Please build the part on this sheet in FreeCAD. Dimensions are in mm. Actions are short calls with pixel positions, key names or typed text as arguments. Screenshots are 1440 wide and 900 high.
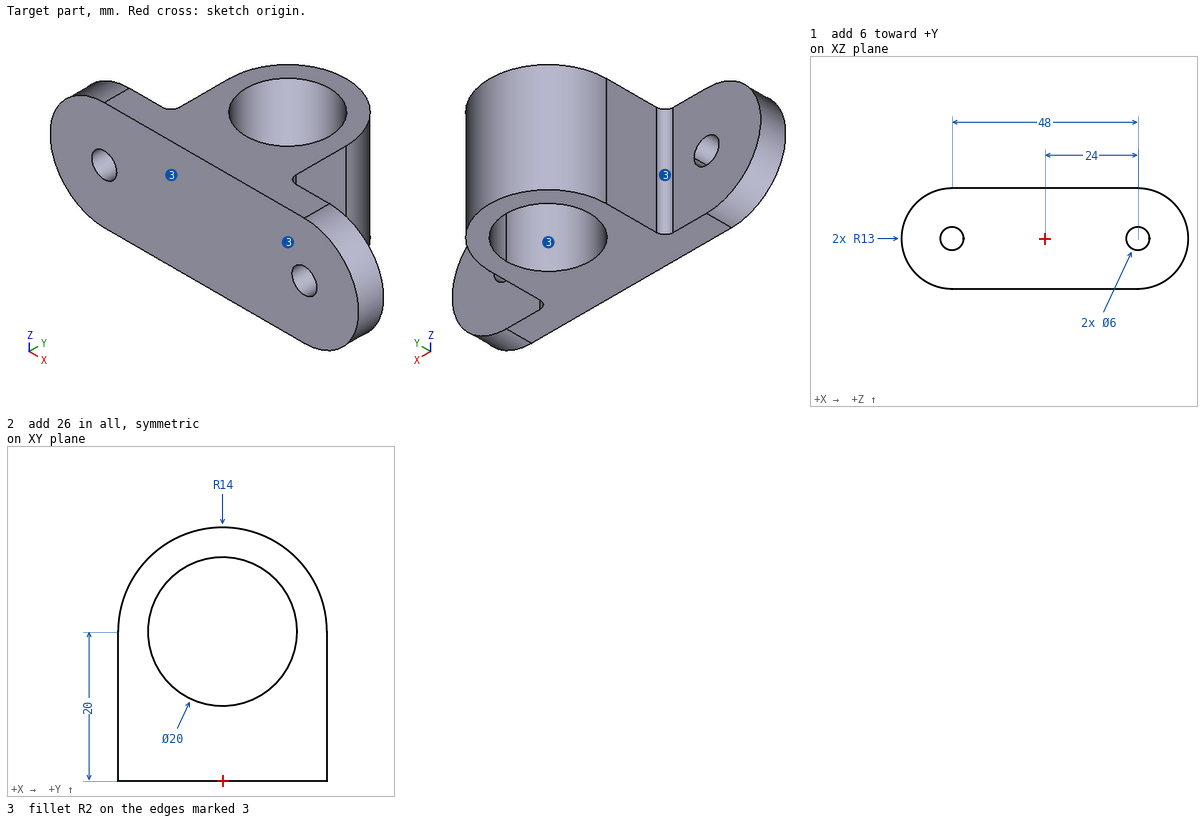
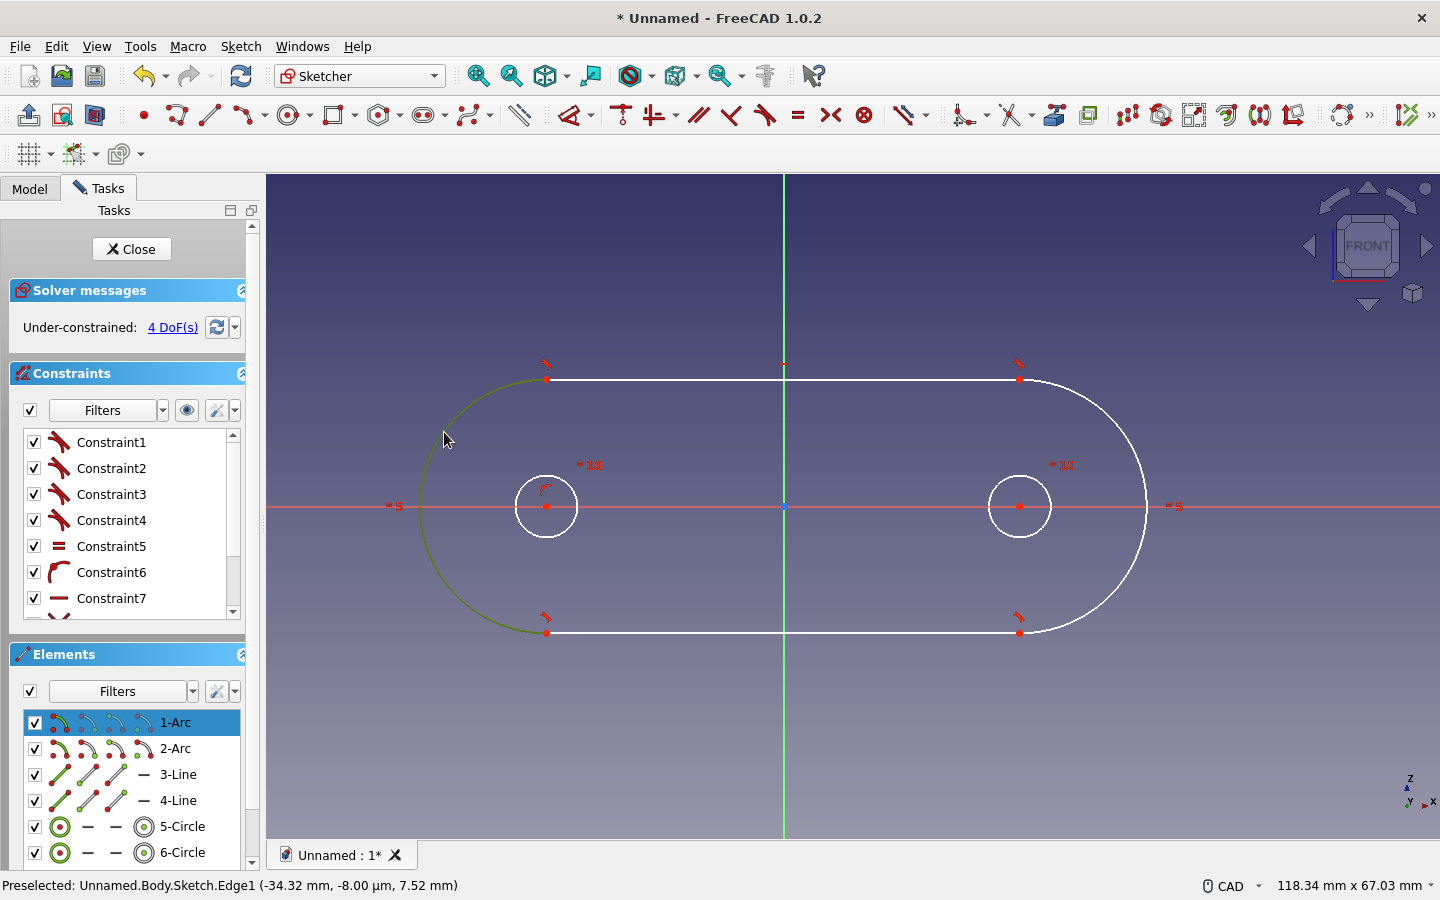
key(k)
key(r)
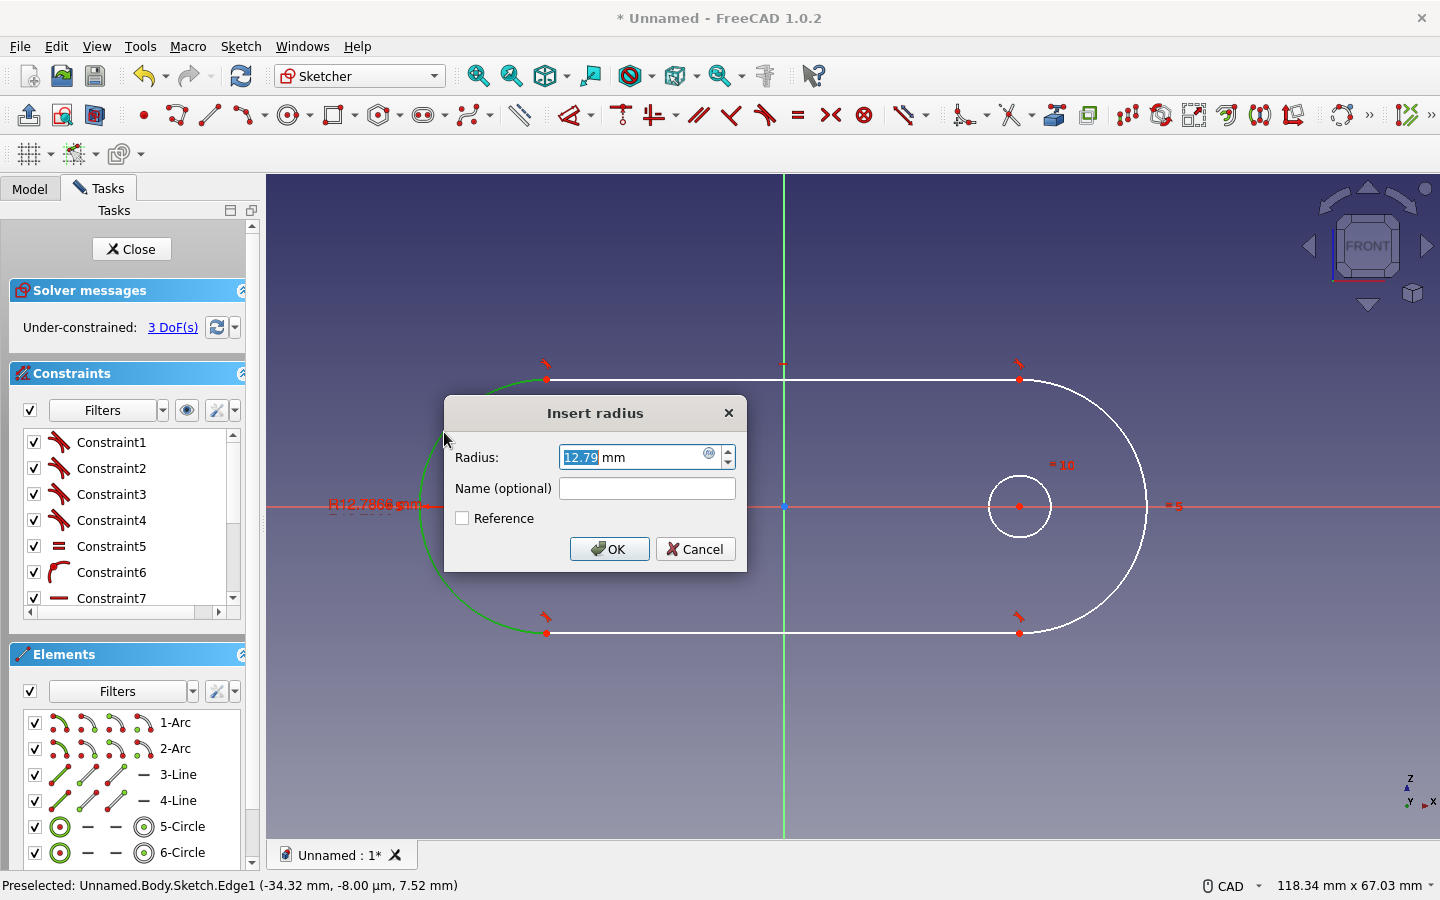
text(13)
key(Return)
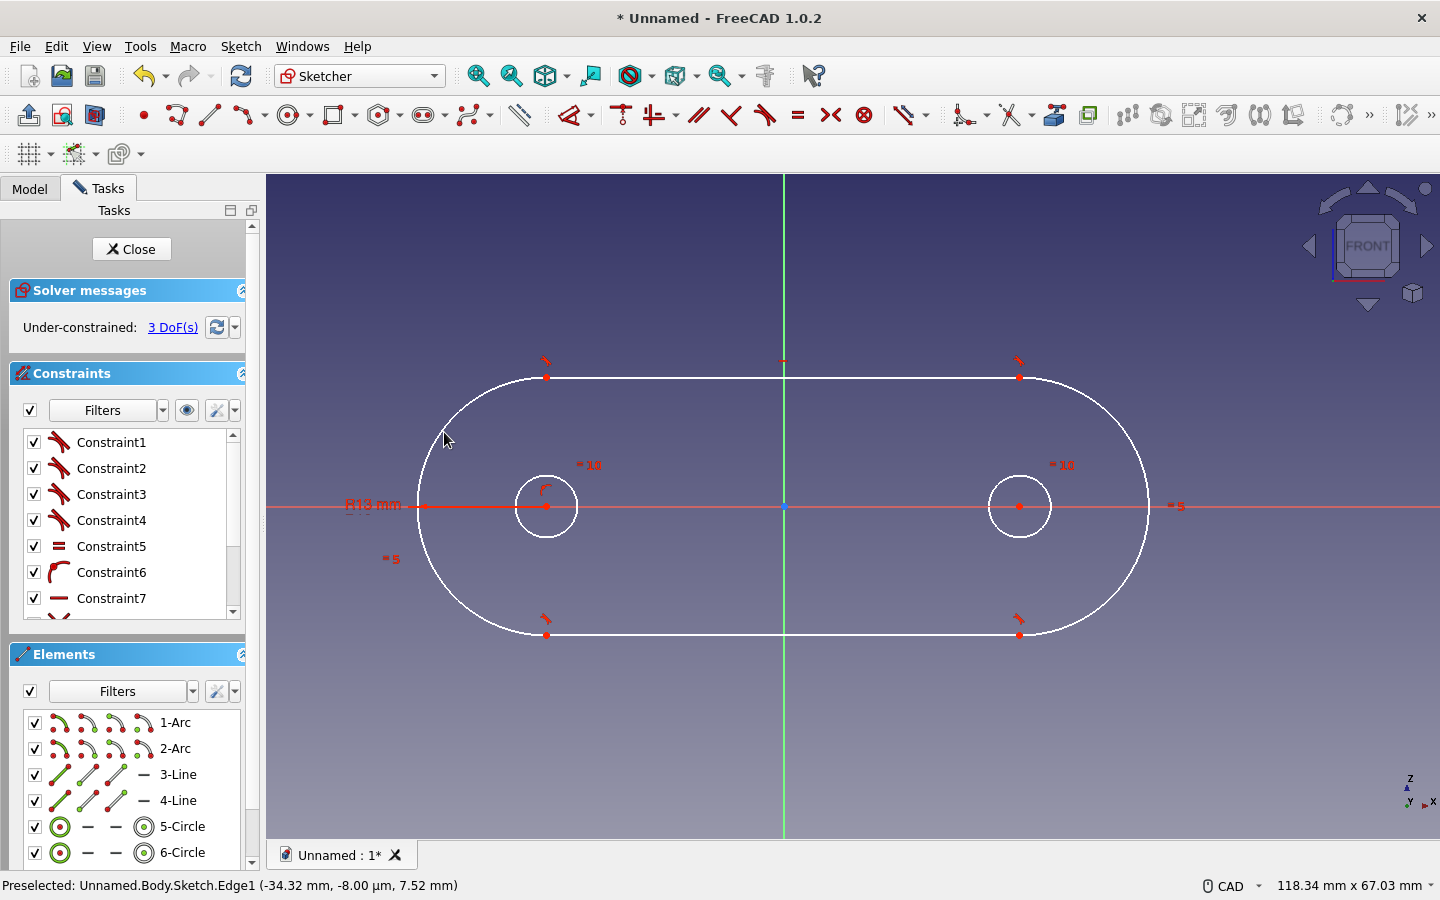
click(1042, 485)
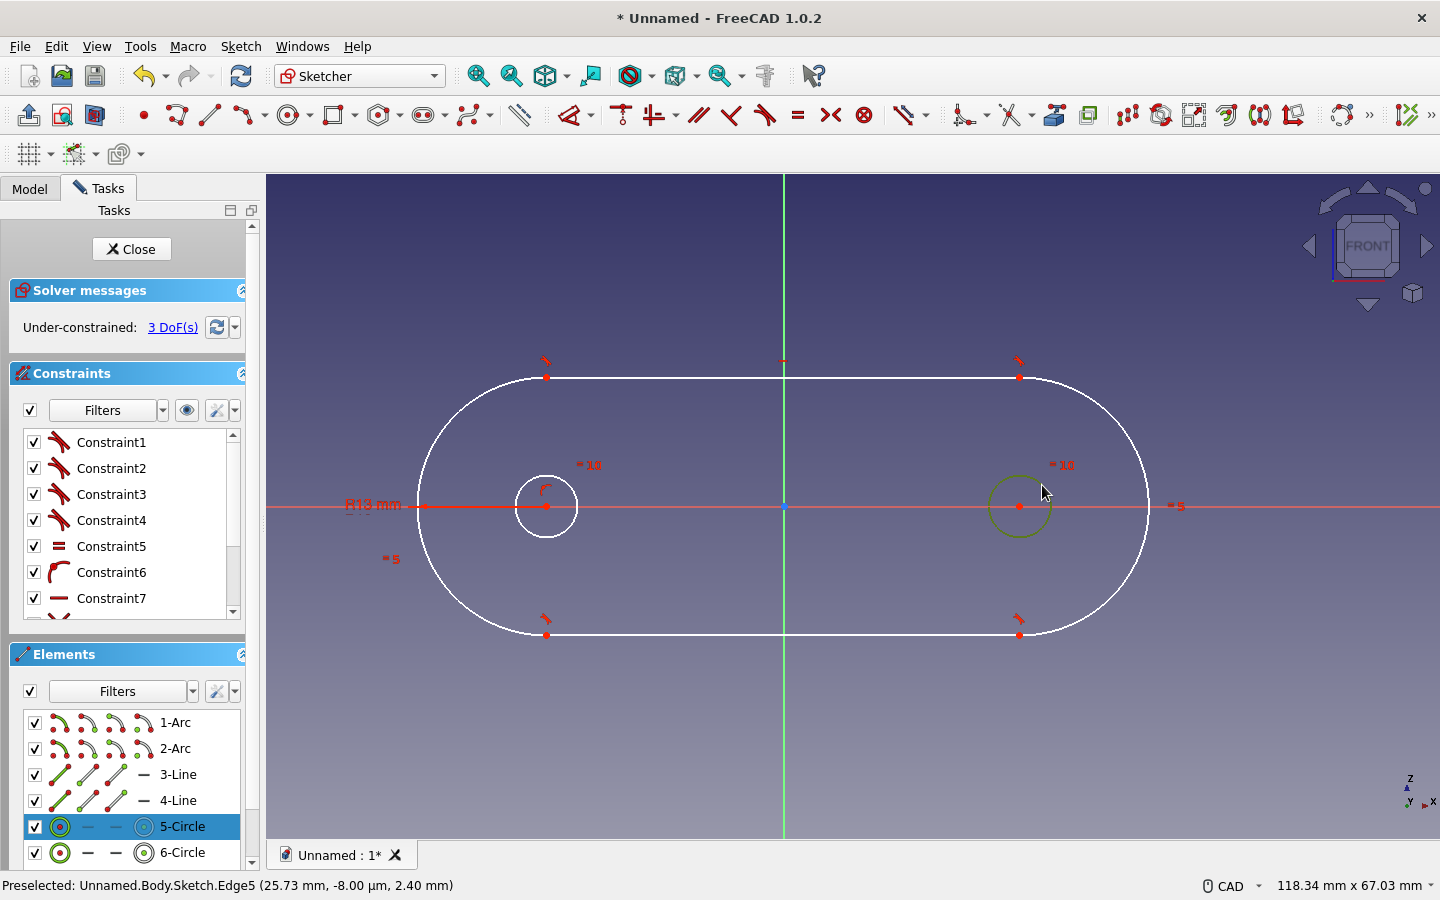
key(k)
key(o)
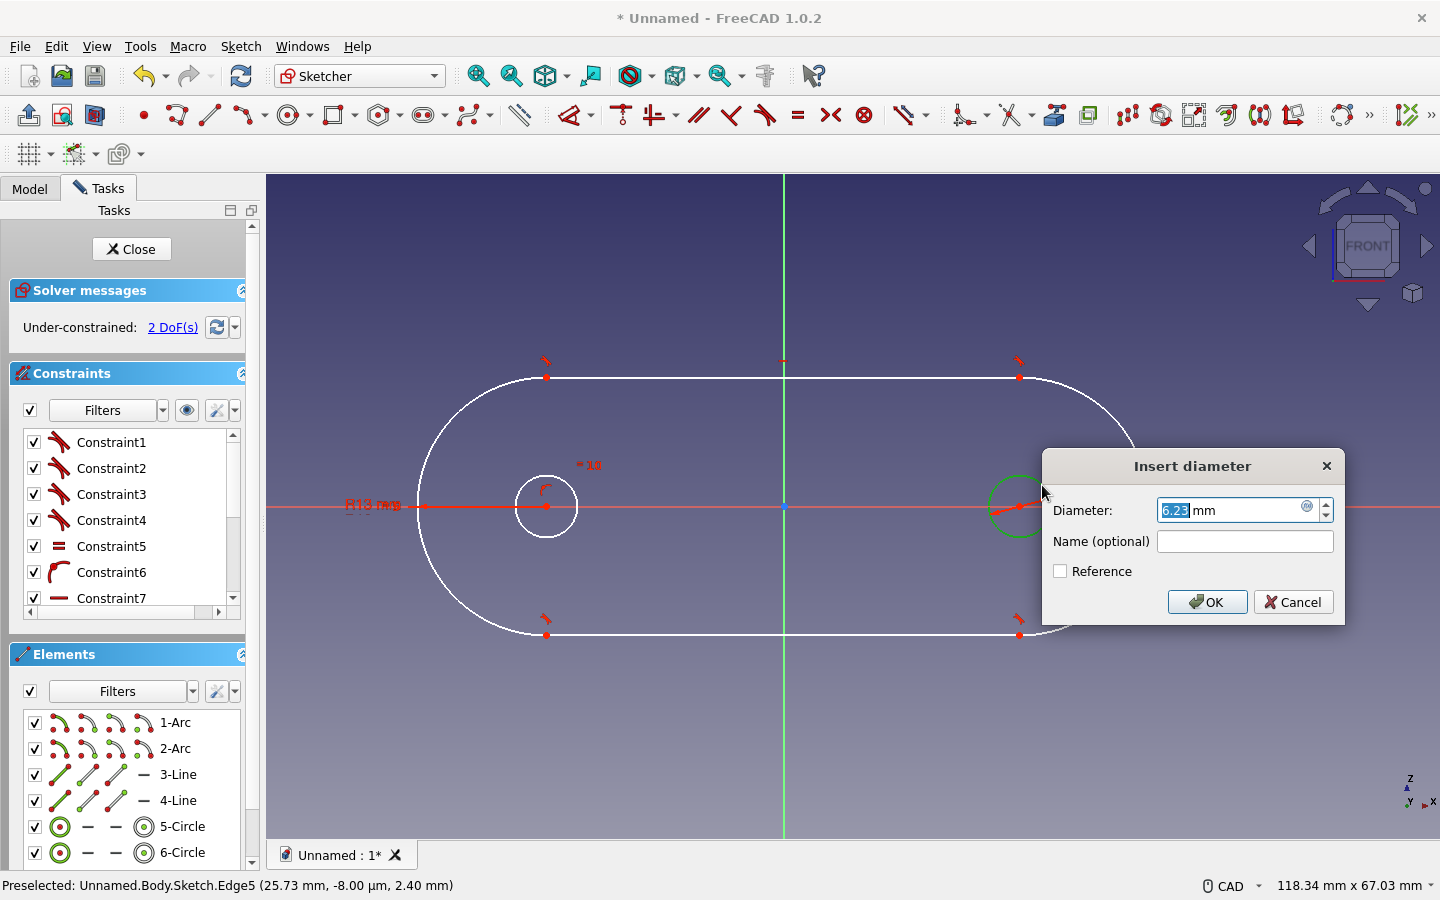
text(6)
key(Return)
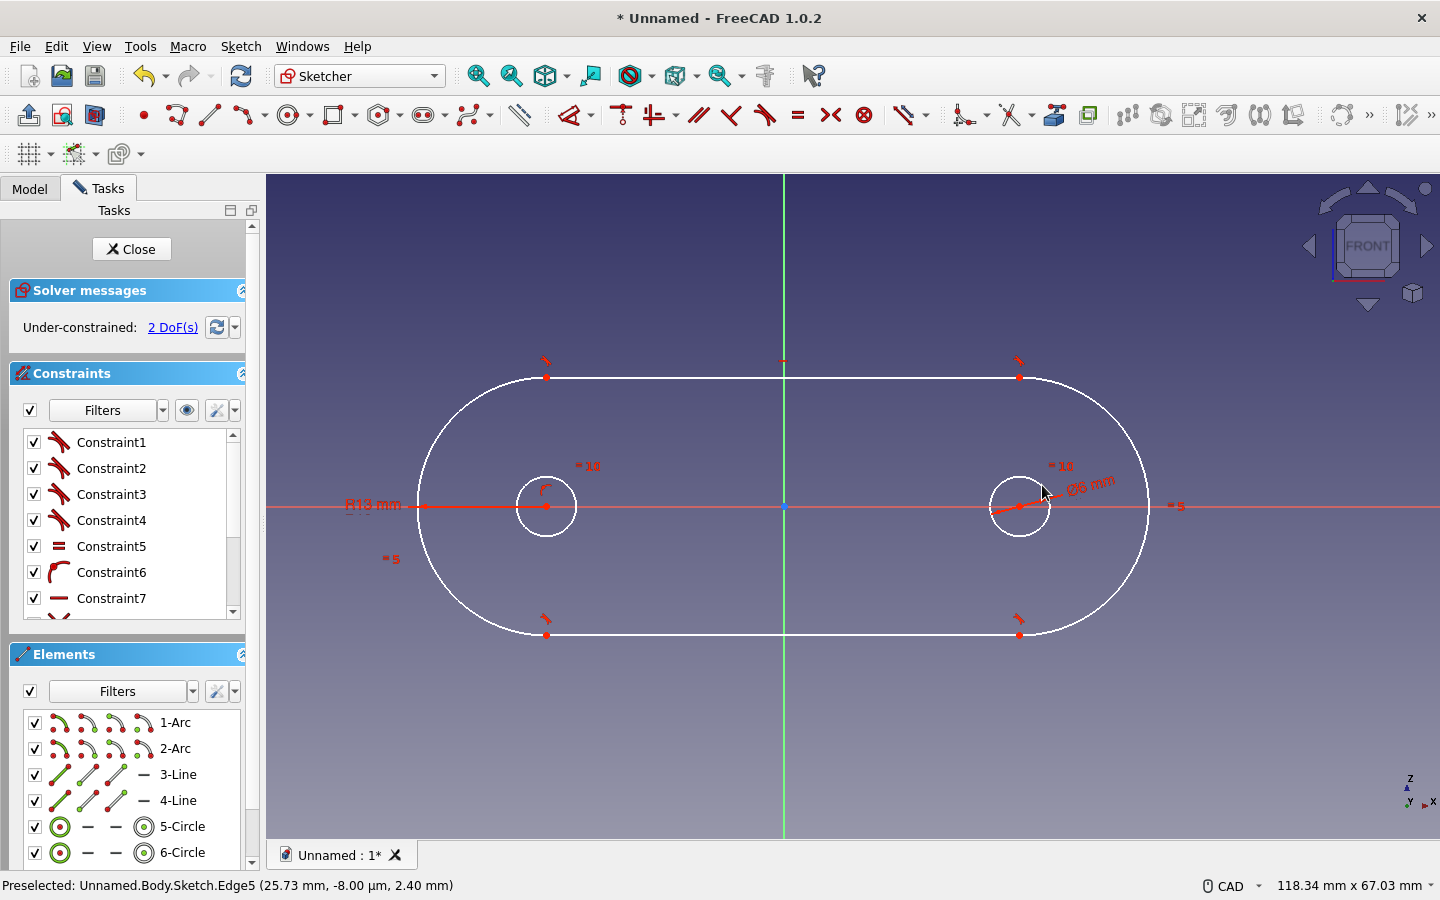
click(689, 378)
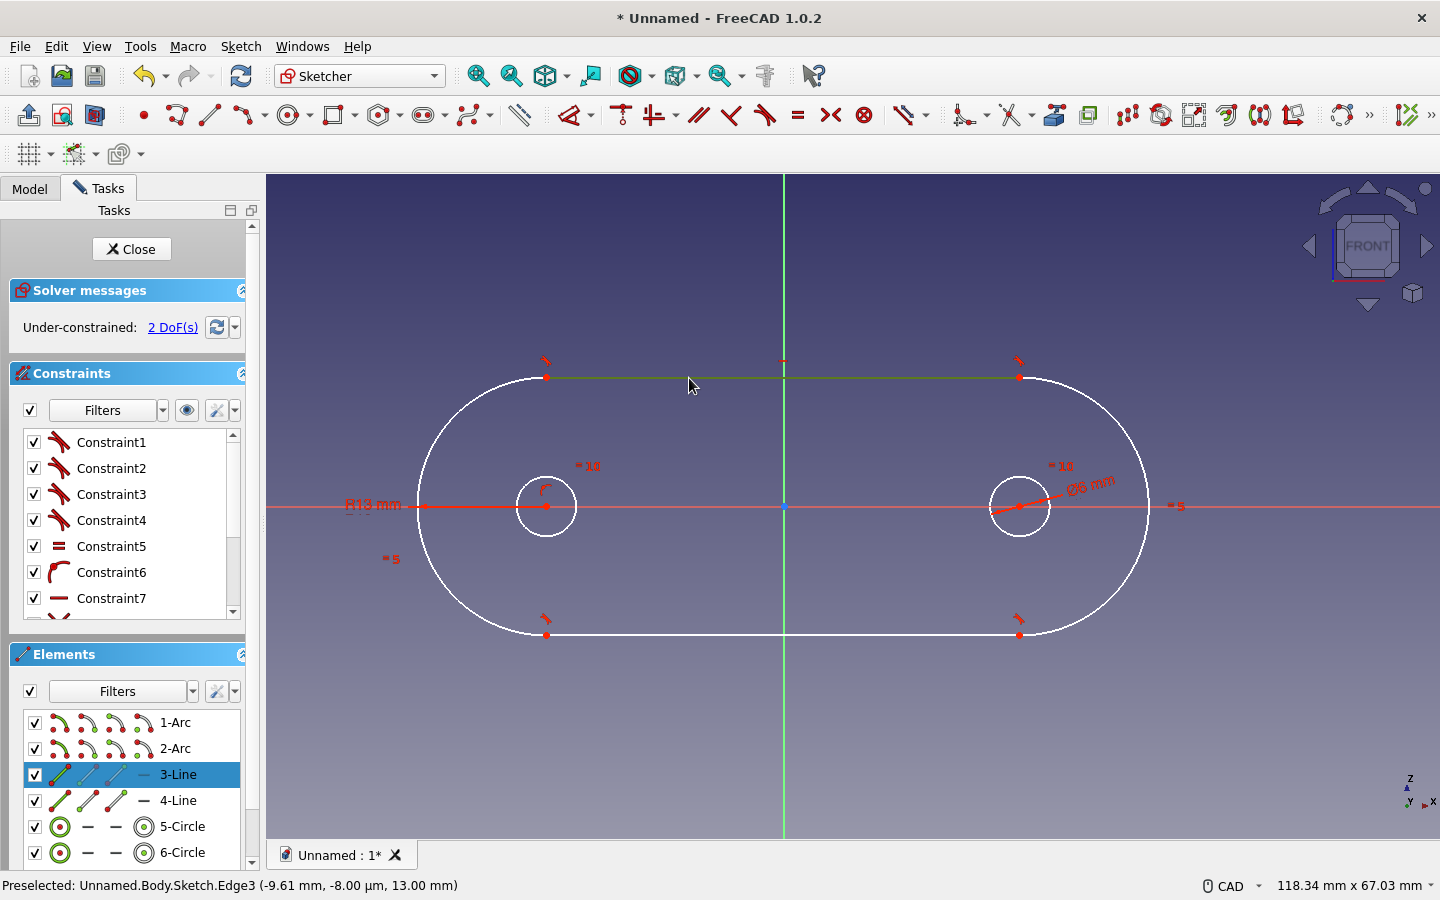
key(l)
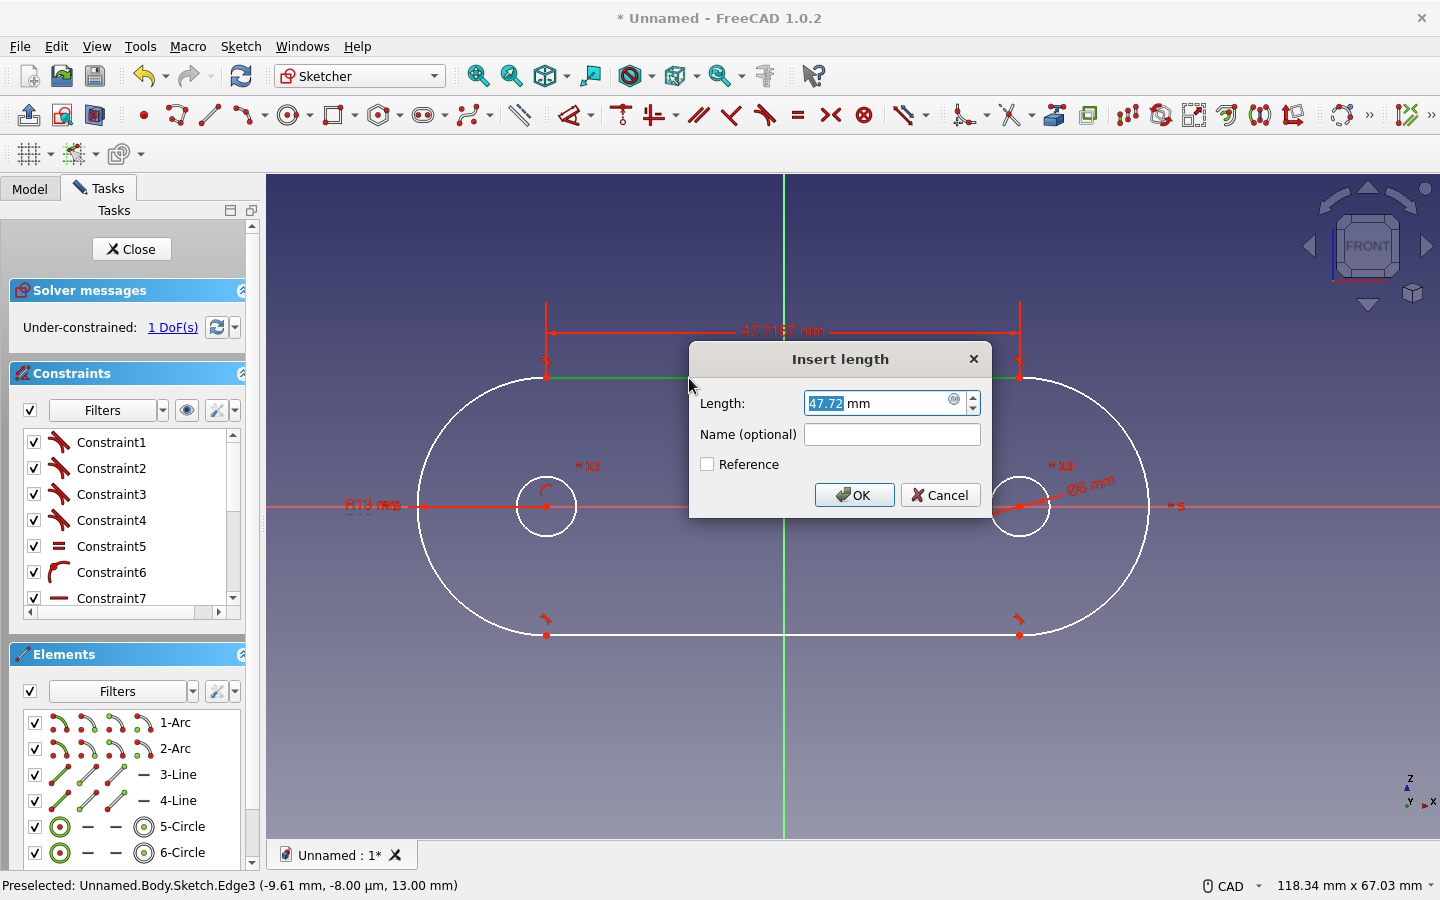
text(48)
key(Return)